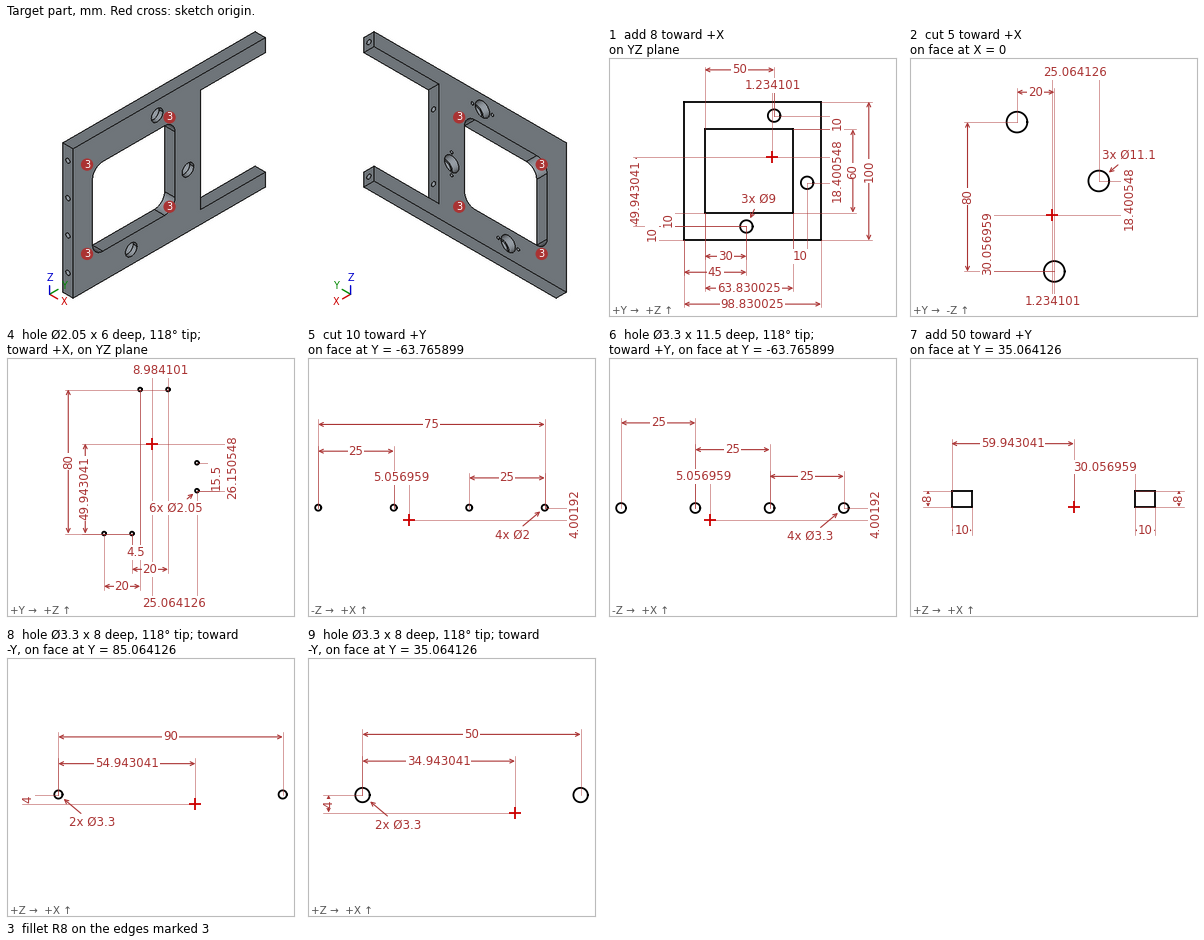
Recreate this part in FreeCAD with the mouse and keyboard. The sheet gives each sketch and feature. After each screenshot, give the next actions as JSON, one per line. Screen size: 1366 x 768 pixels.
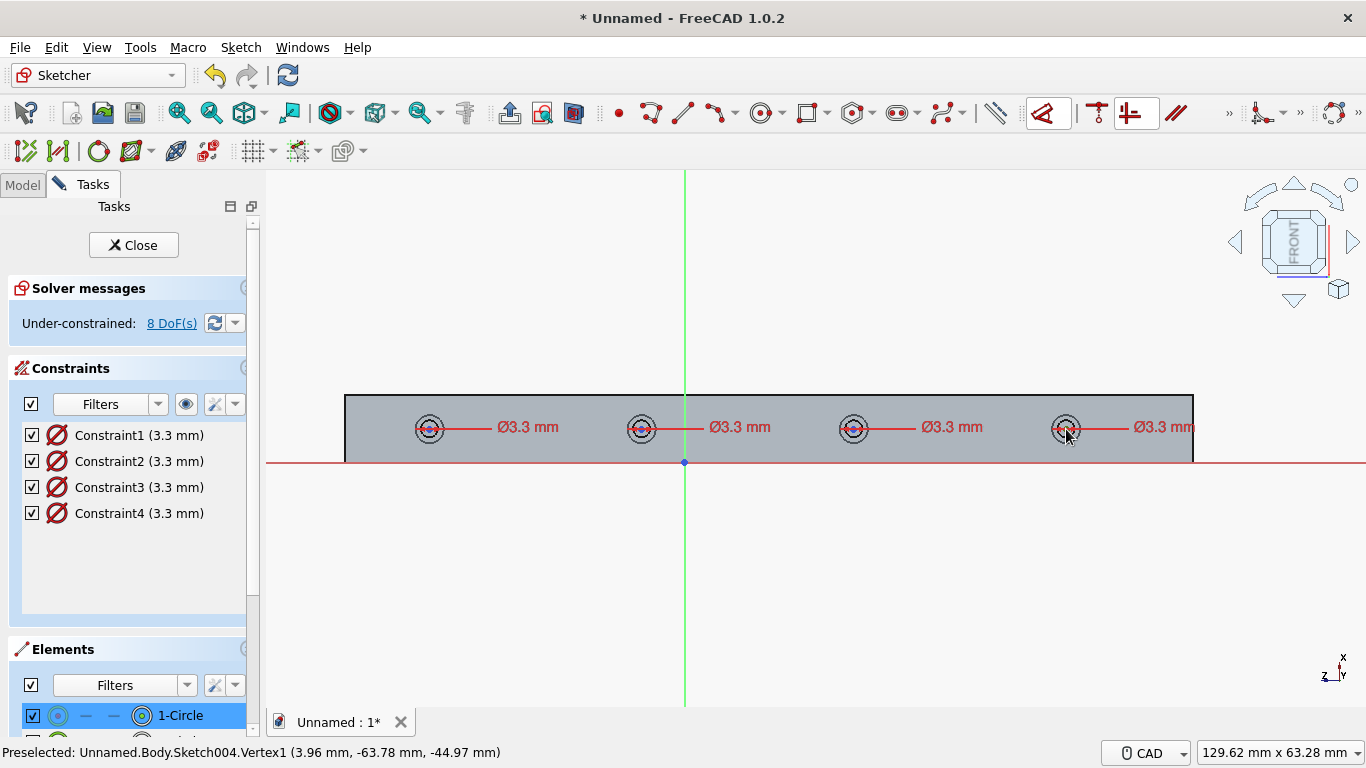
{"action": "left_click", "coordinate": [854, 429]}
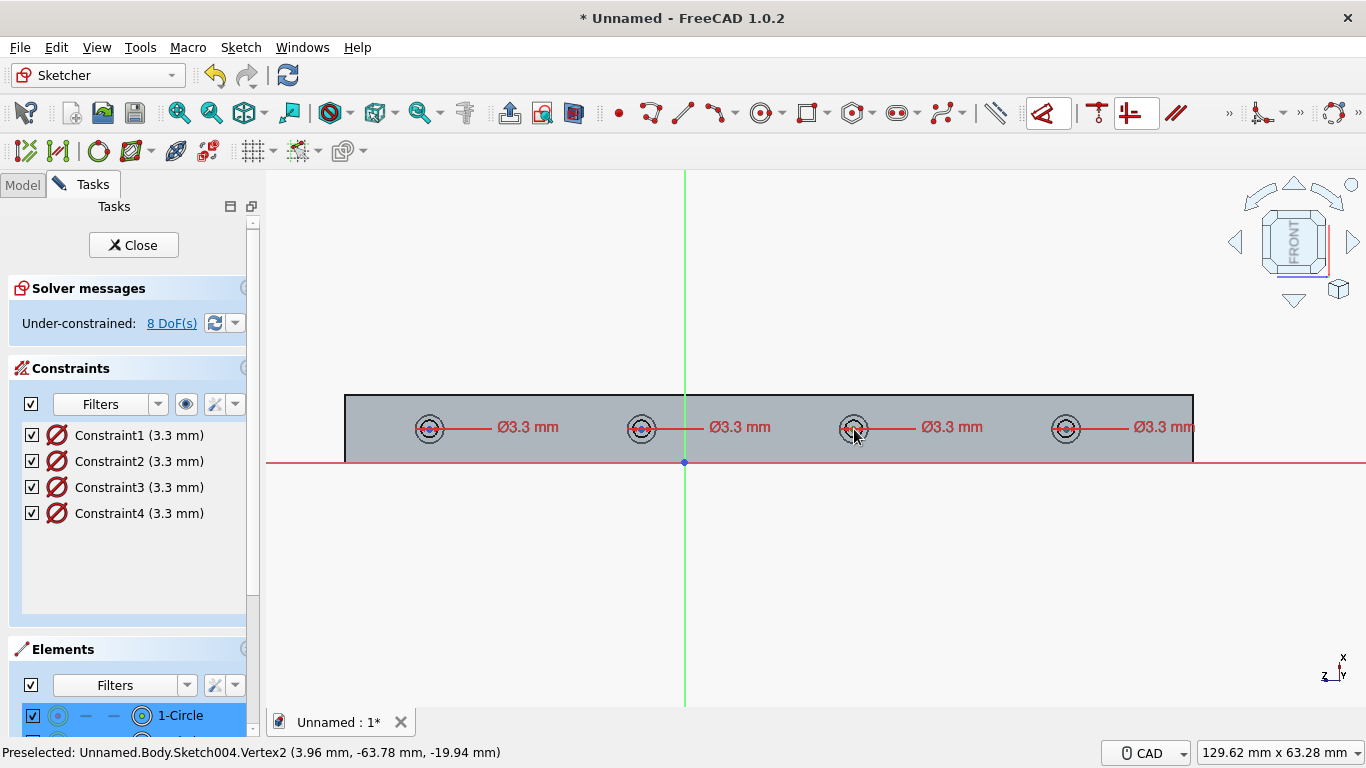
{"action": "left_click", "coordinate": [1154, 114]}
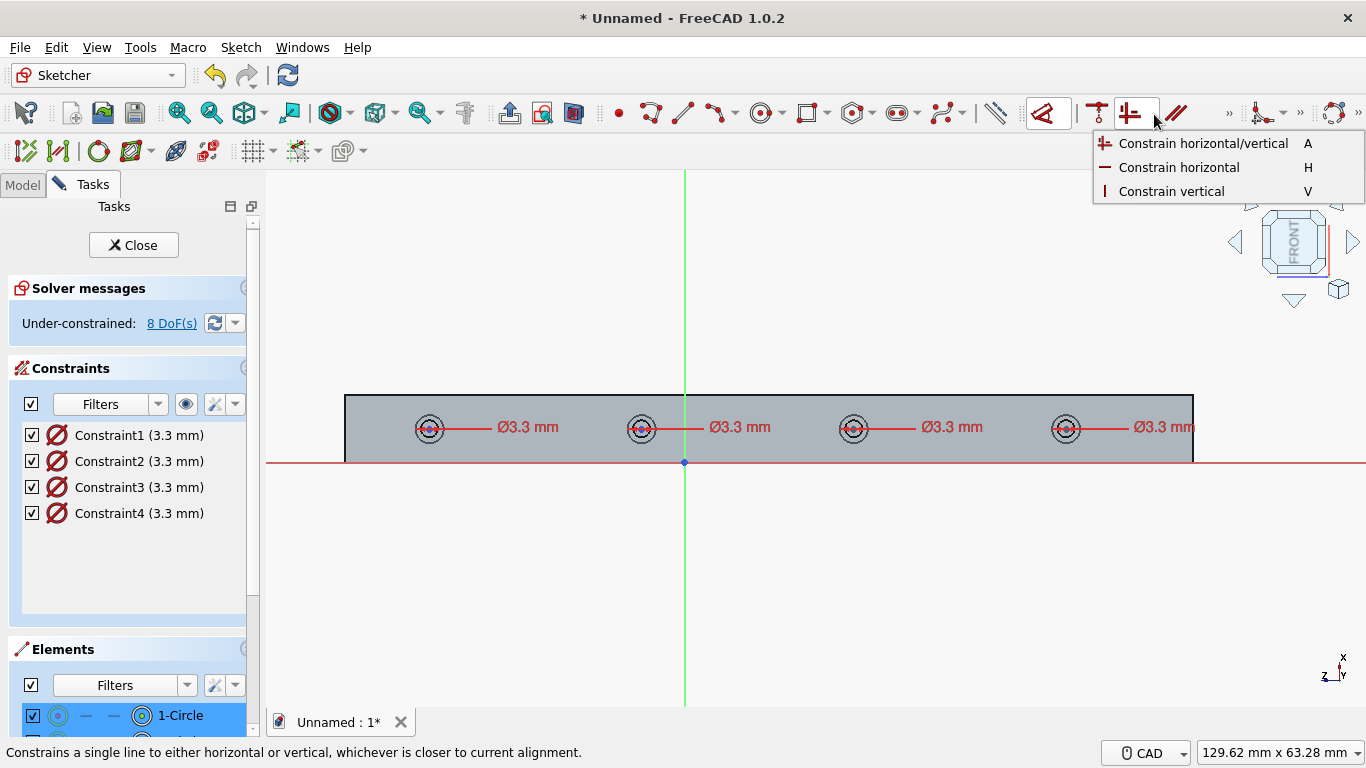
{"action": "left_click", "coordinate": [1229, 167]}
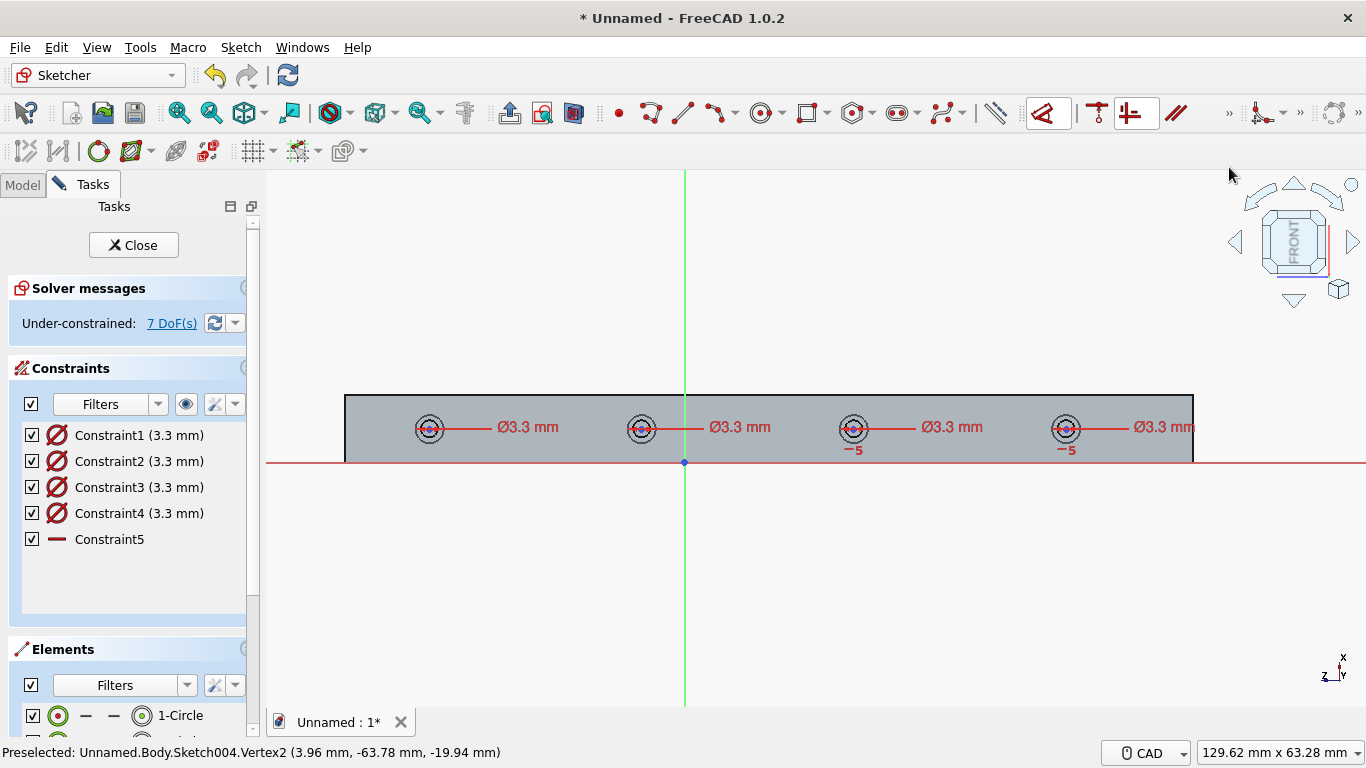
{"action": "left_click", "coordinate": [854, 429]}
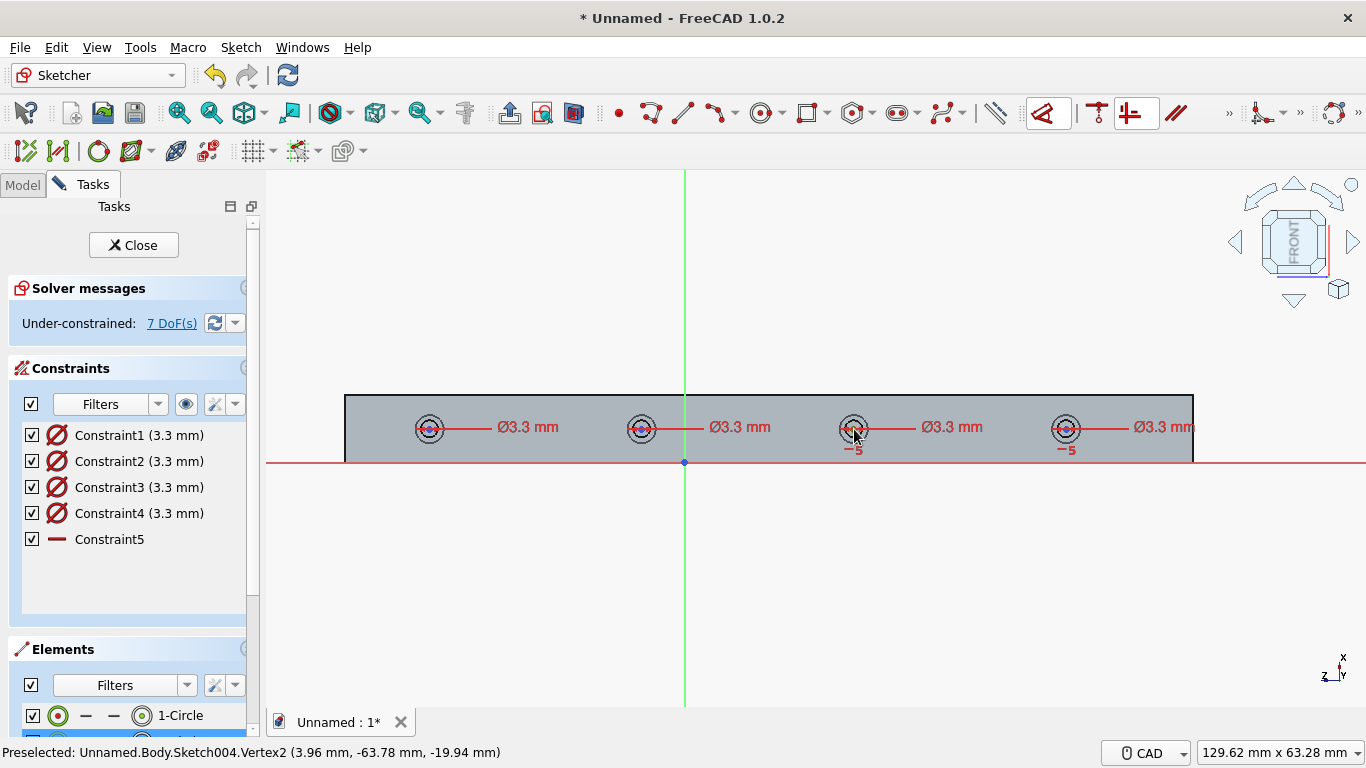
{"action": "left_click", "coordinate": [642, 429]}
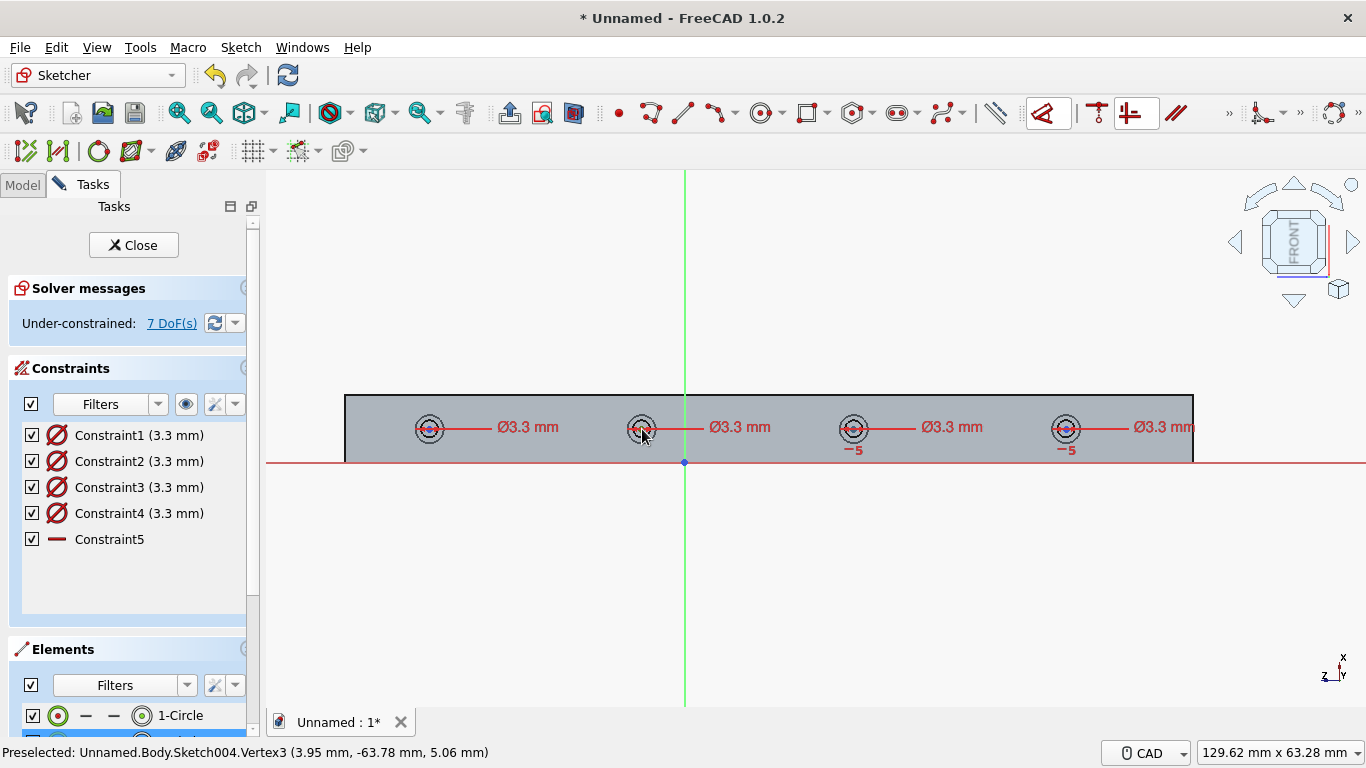
{"action": "key", "text": "h"}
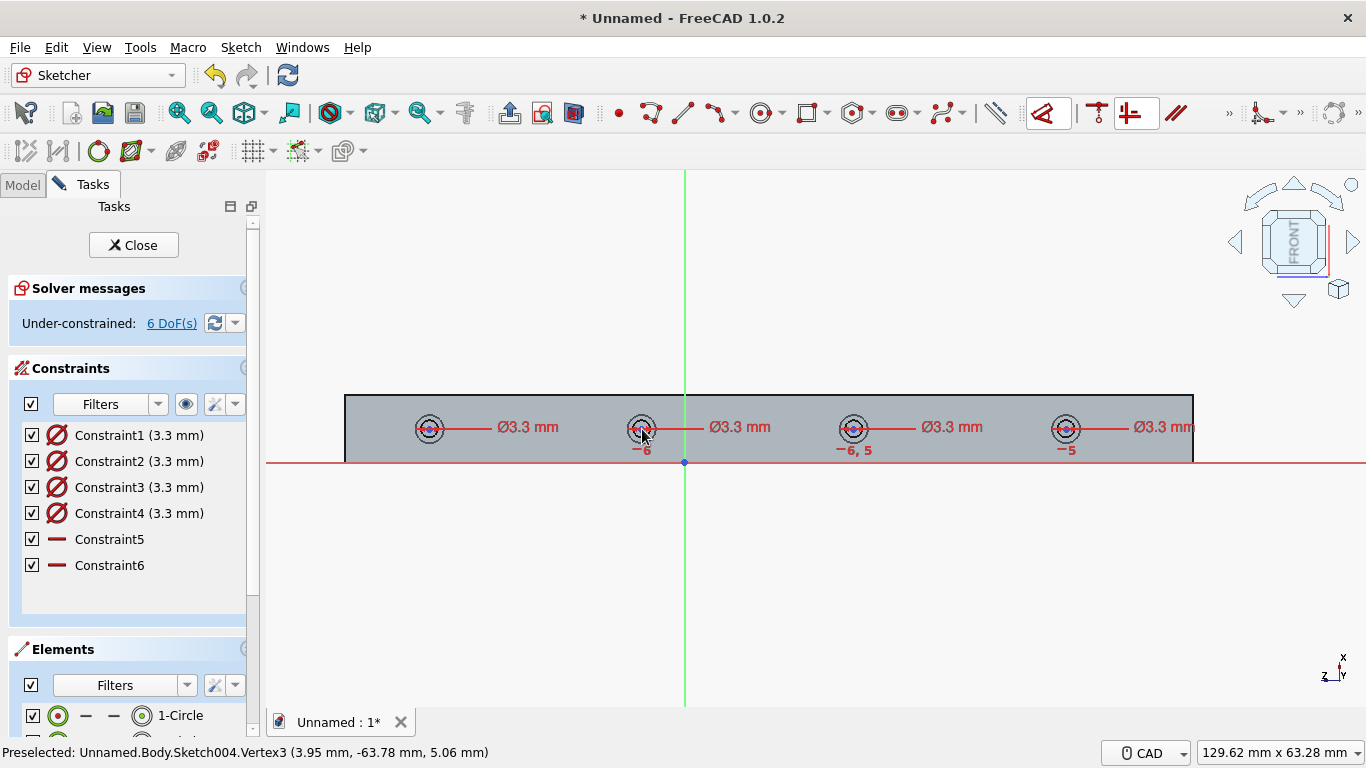
{"action": "left_click", "coordinate": [642, 429]}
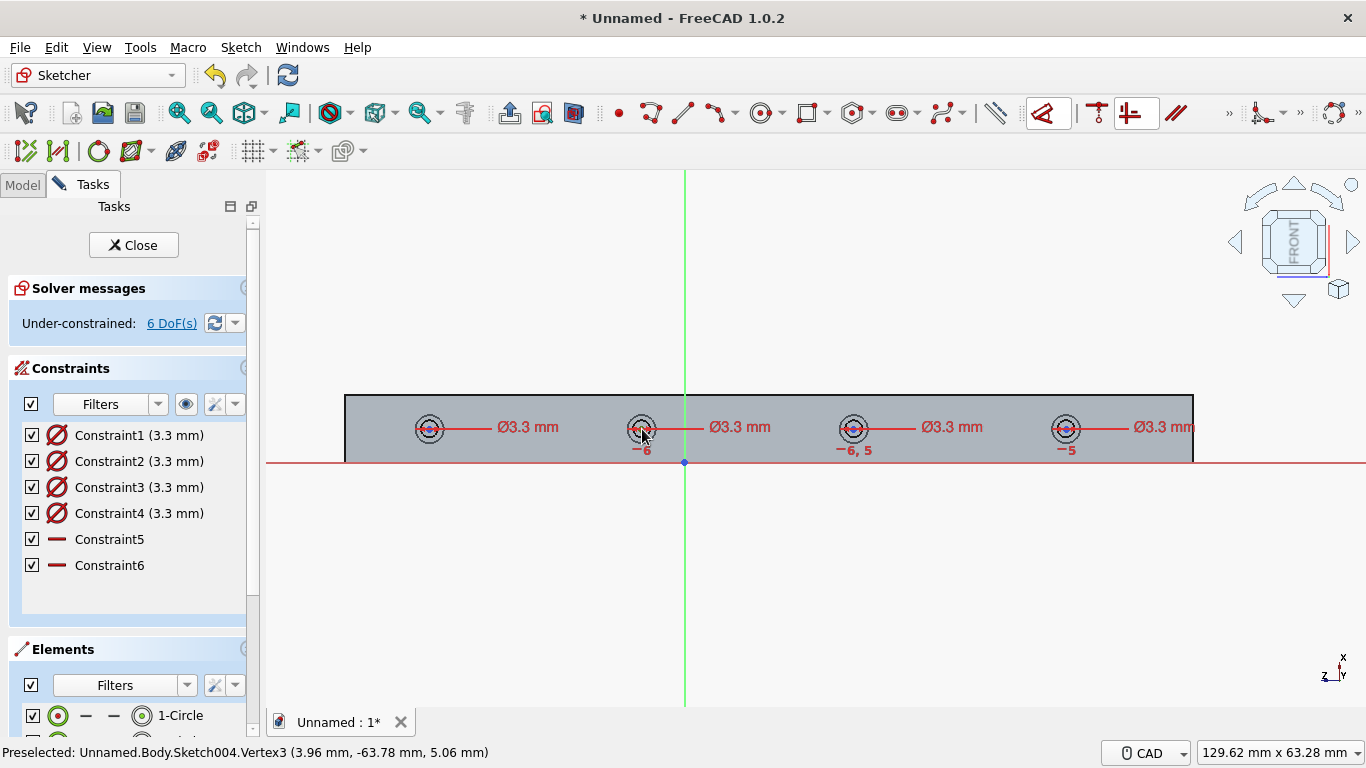
{"action": "left_click", "coordinate": [430, 429]}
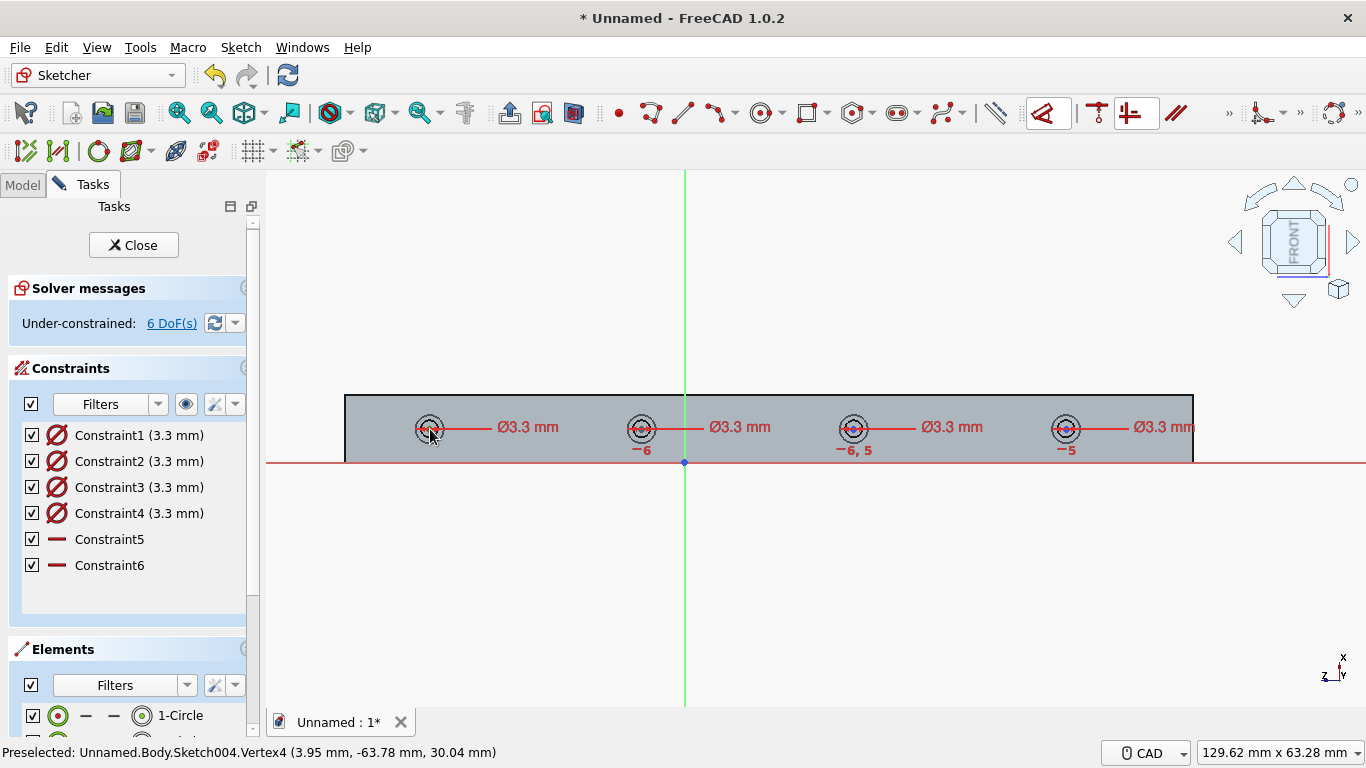
{"action": "key", "text": "h"}